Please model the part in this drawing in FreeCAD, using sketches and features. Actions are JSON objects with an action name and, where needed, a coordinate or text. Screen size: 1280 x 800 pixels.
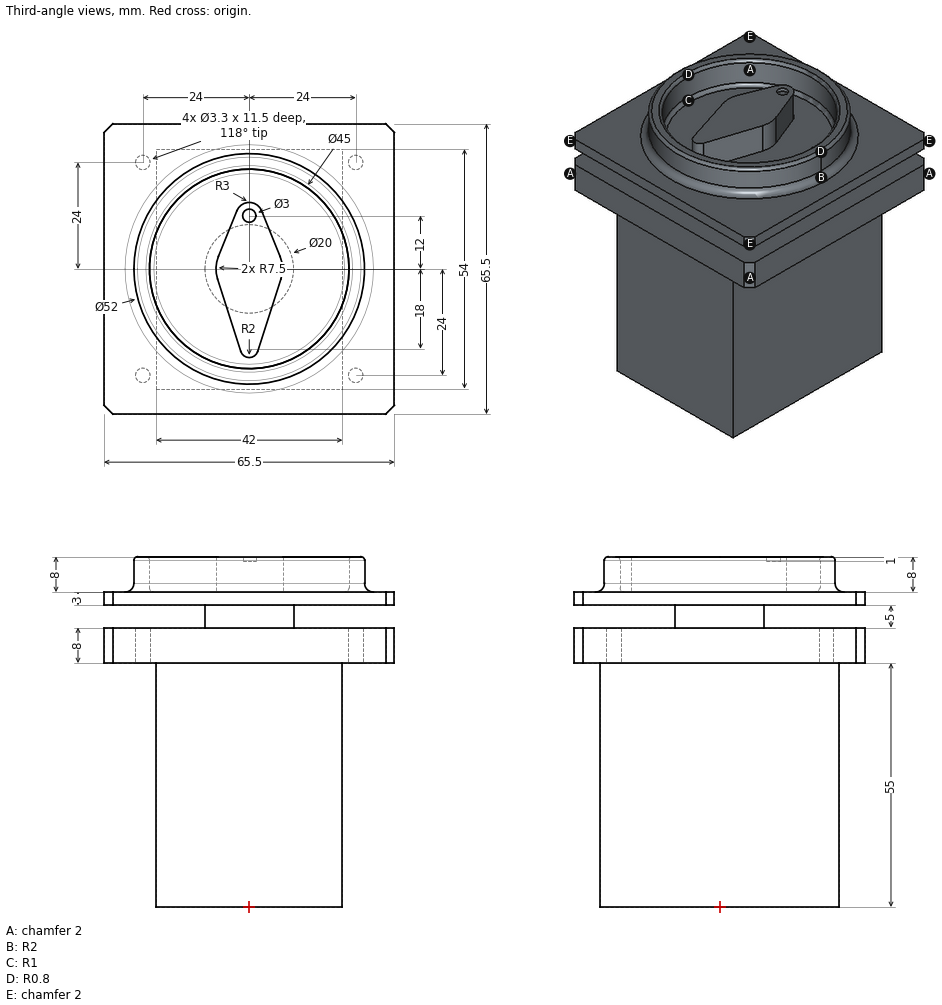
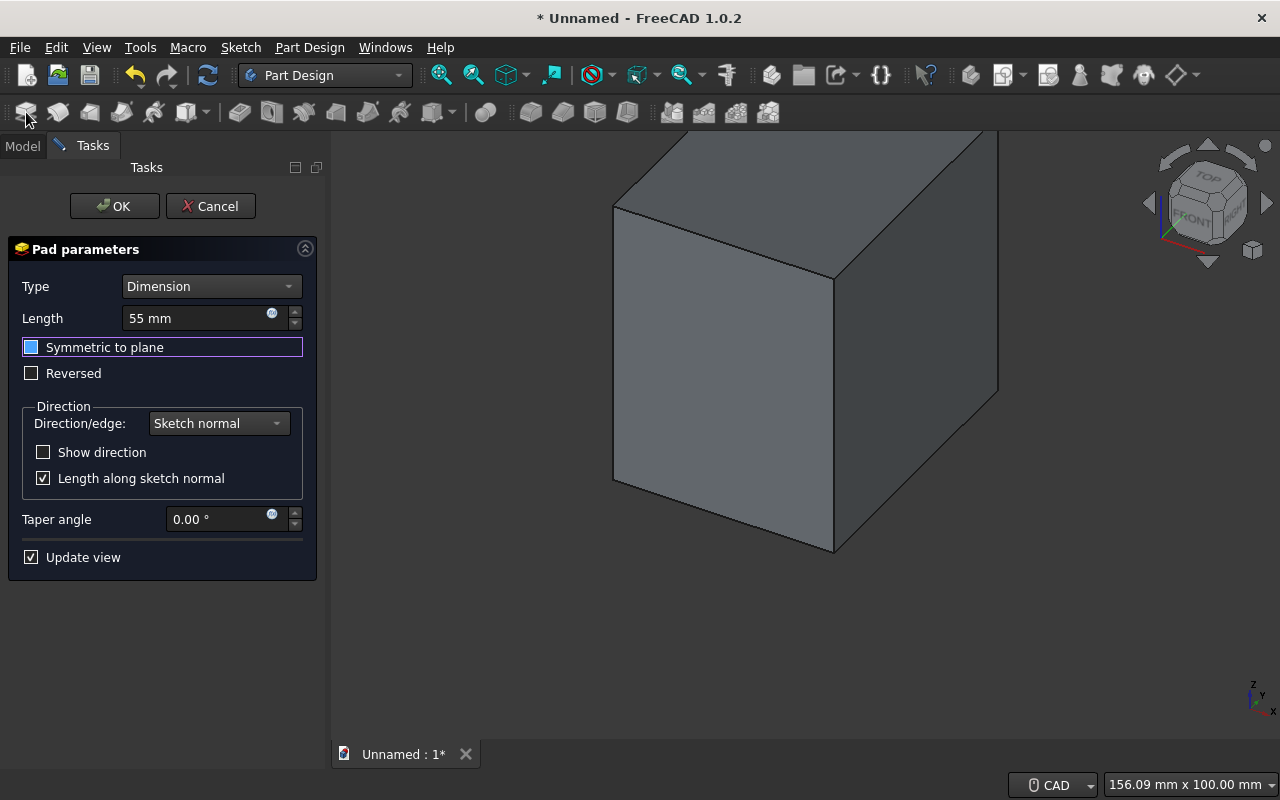
{"action": "left_click", "coordinate": [115, 206]}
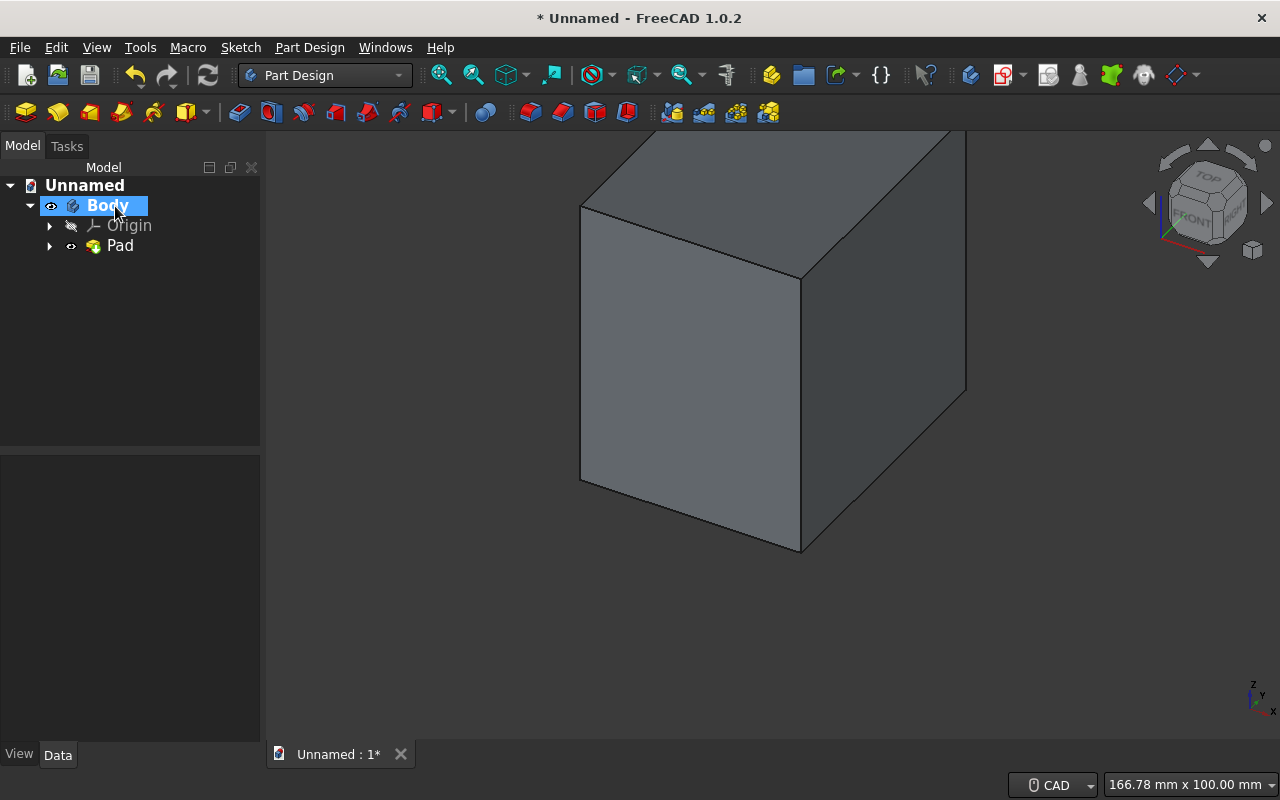
{"action": "left_click", "coordinate": [442, 76]}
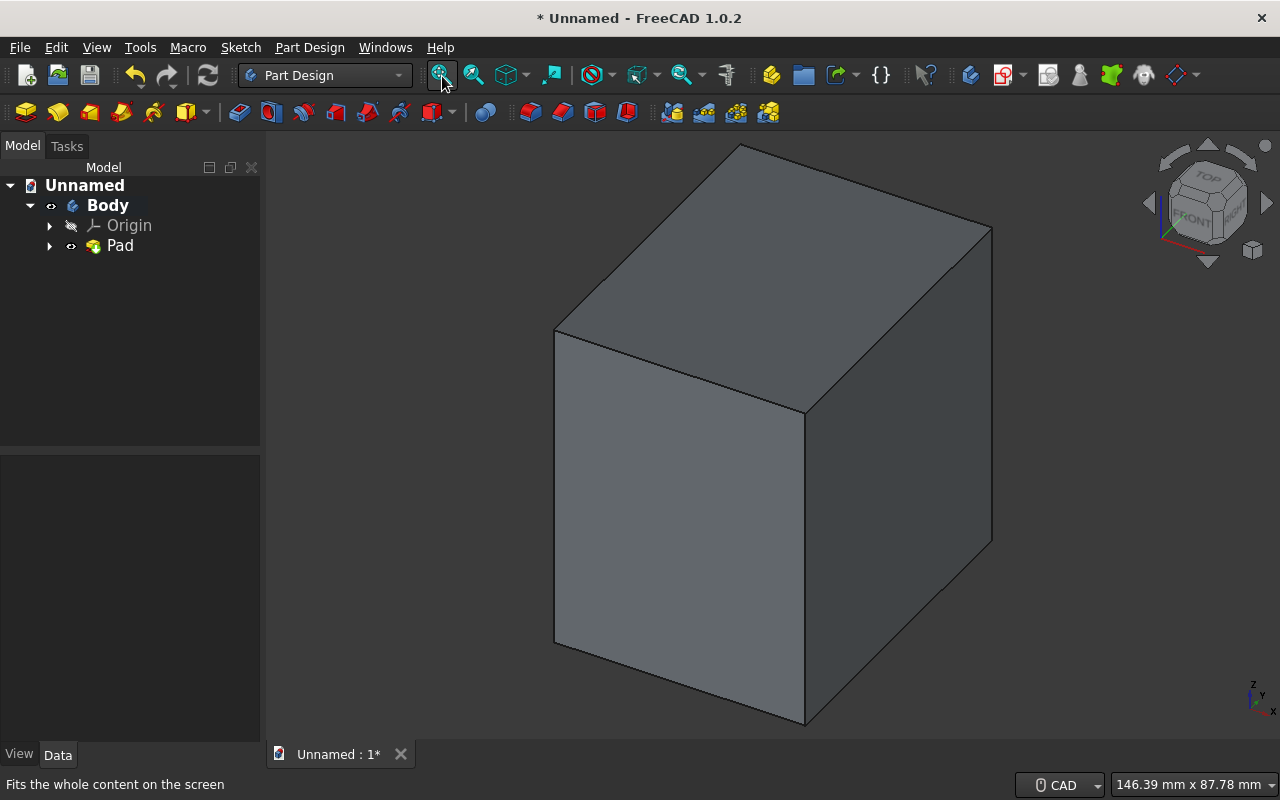
{"action": "left_click", "coordinate": [773, 278]}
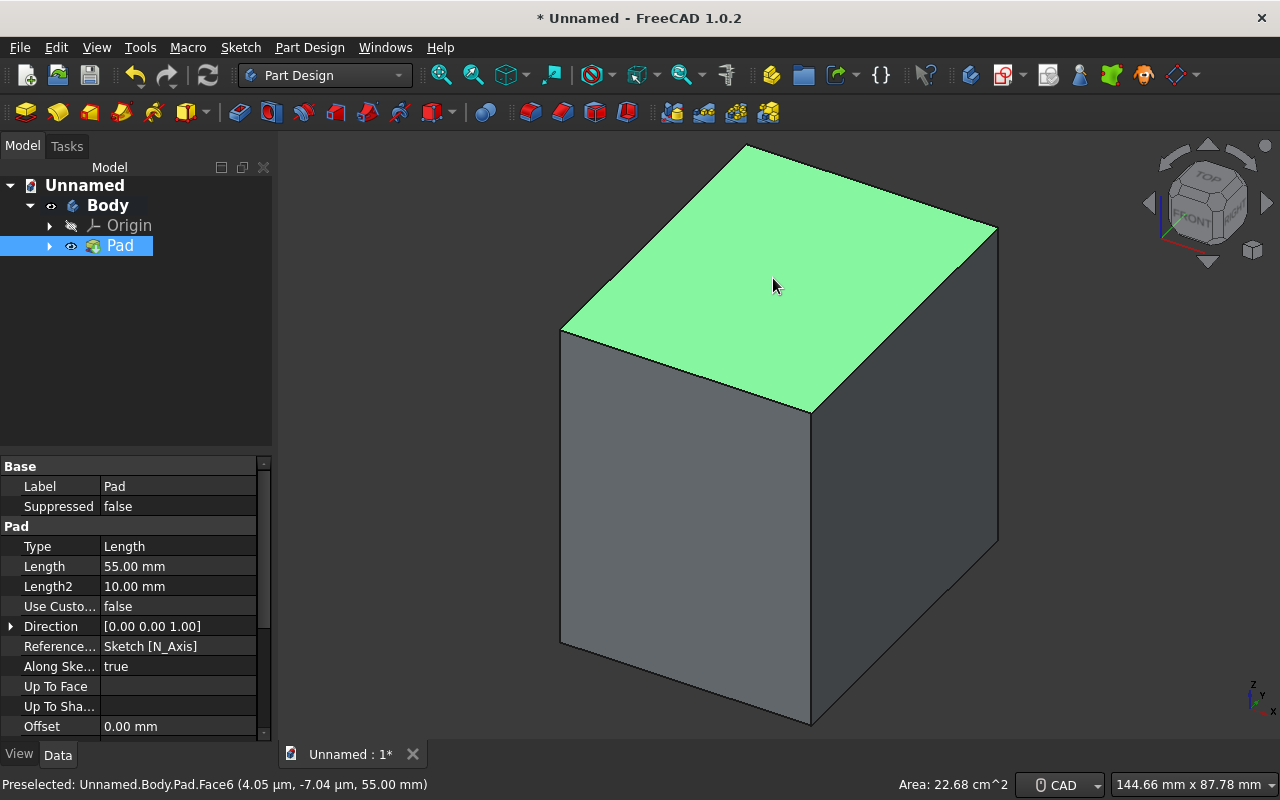
{"action": "left_click", "coordinate": [1004, 76]}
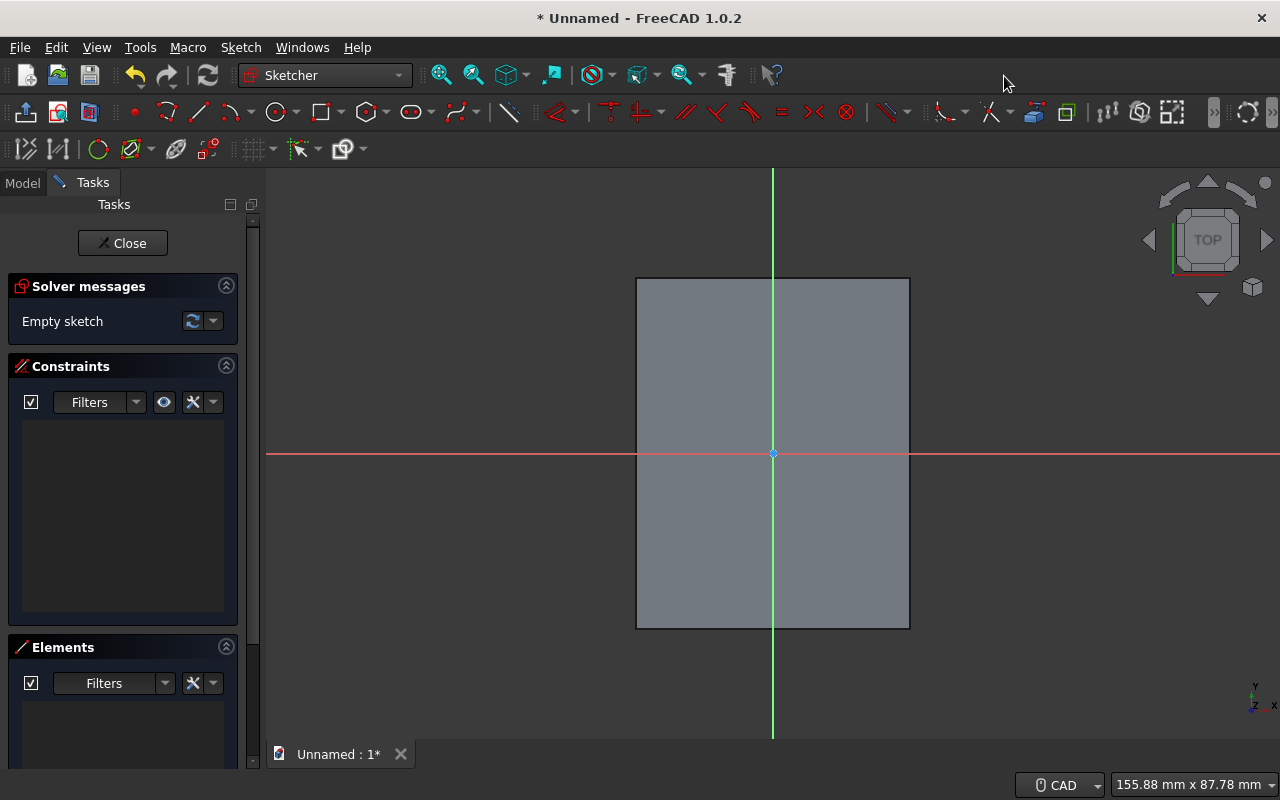
{"action": "left_click", "coordinate": [344, 112]}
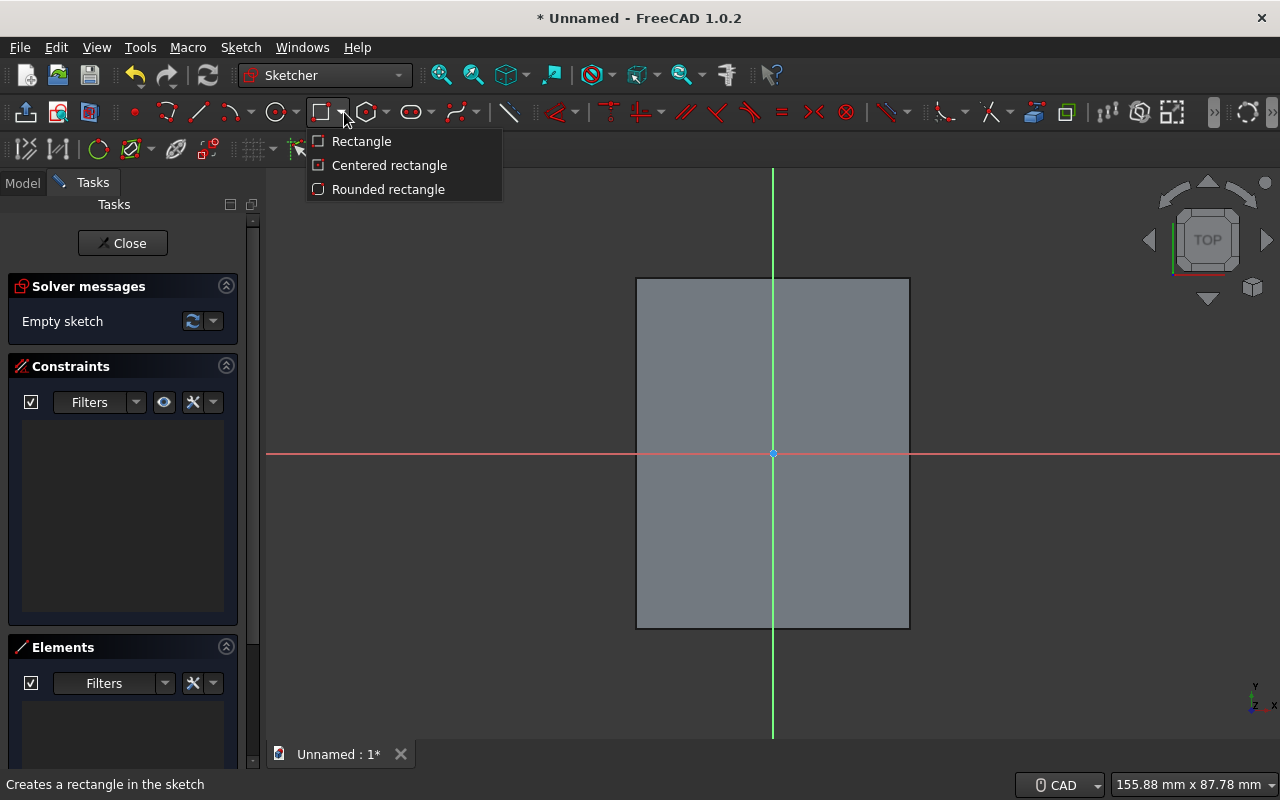
{"action": "left_click", "coordinate": [404, 165]}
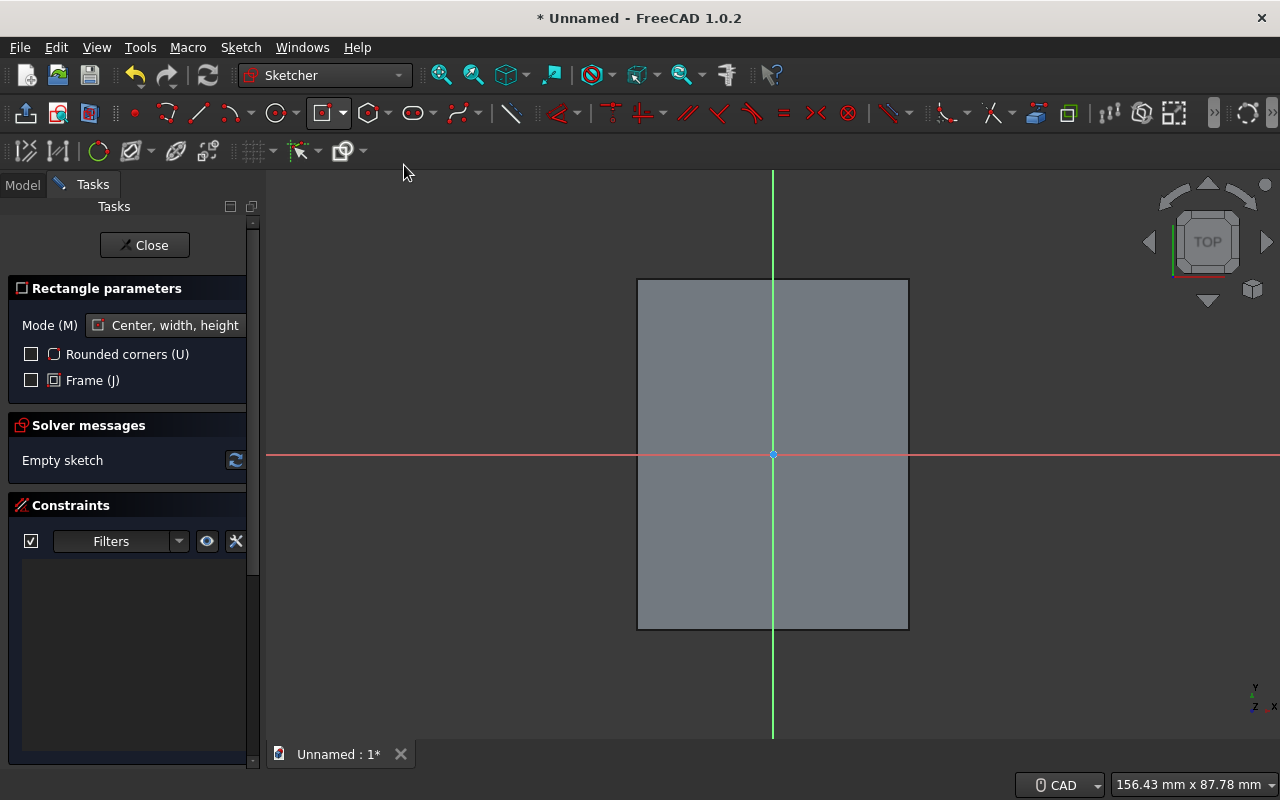
{"action": "left_click", "coordinate": [773, 454]}
{"action": "mouse_move", "coordinate": [985, 242]}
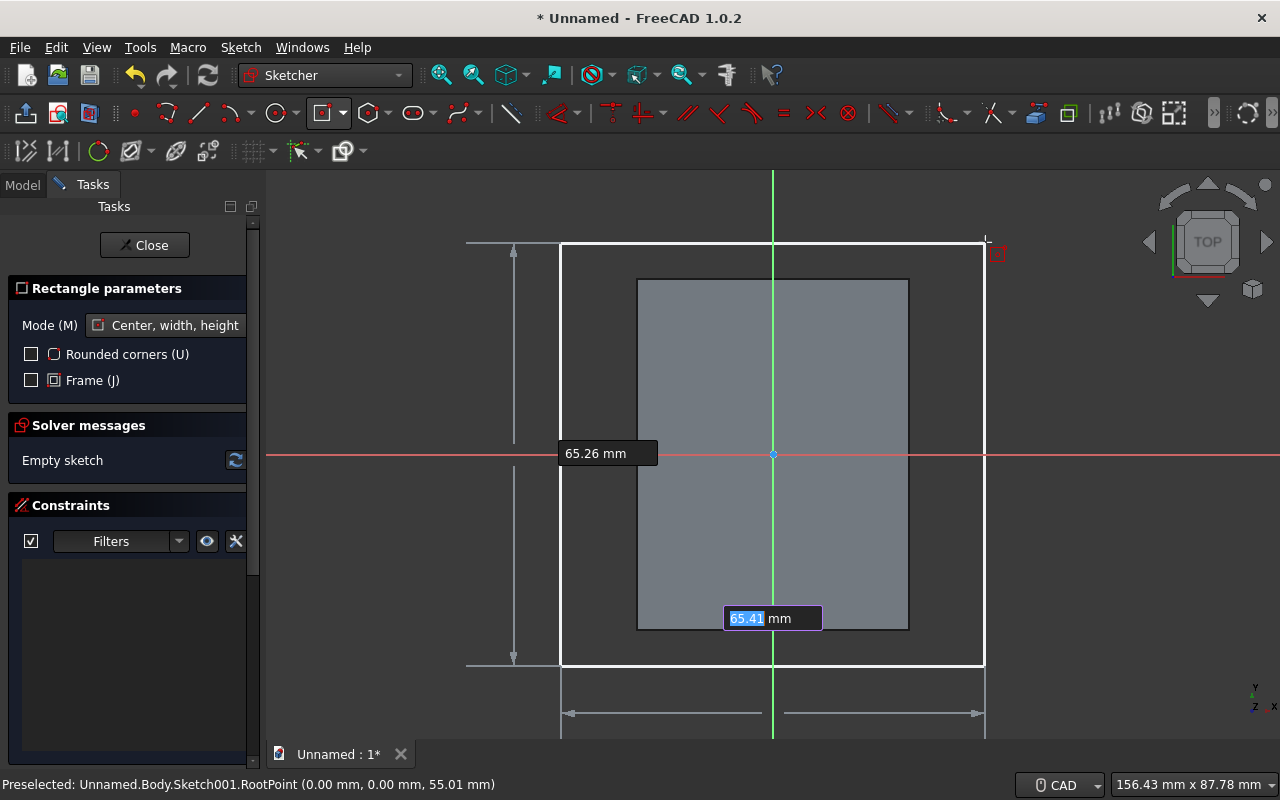
{"action": "type", "text": "65.5"}
{"action": "key", "text": "Tab"}
{"action": "type", "text": "65.5"}
{"action": "key", "text": "Return"}
{"action": "key", "text": "Escape"}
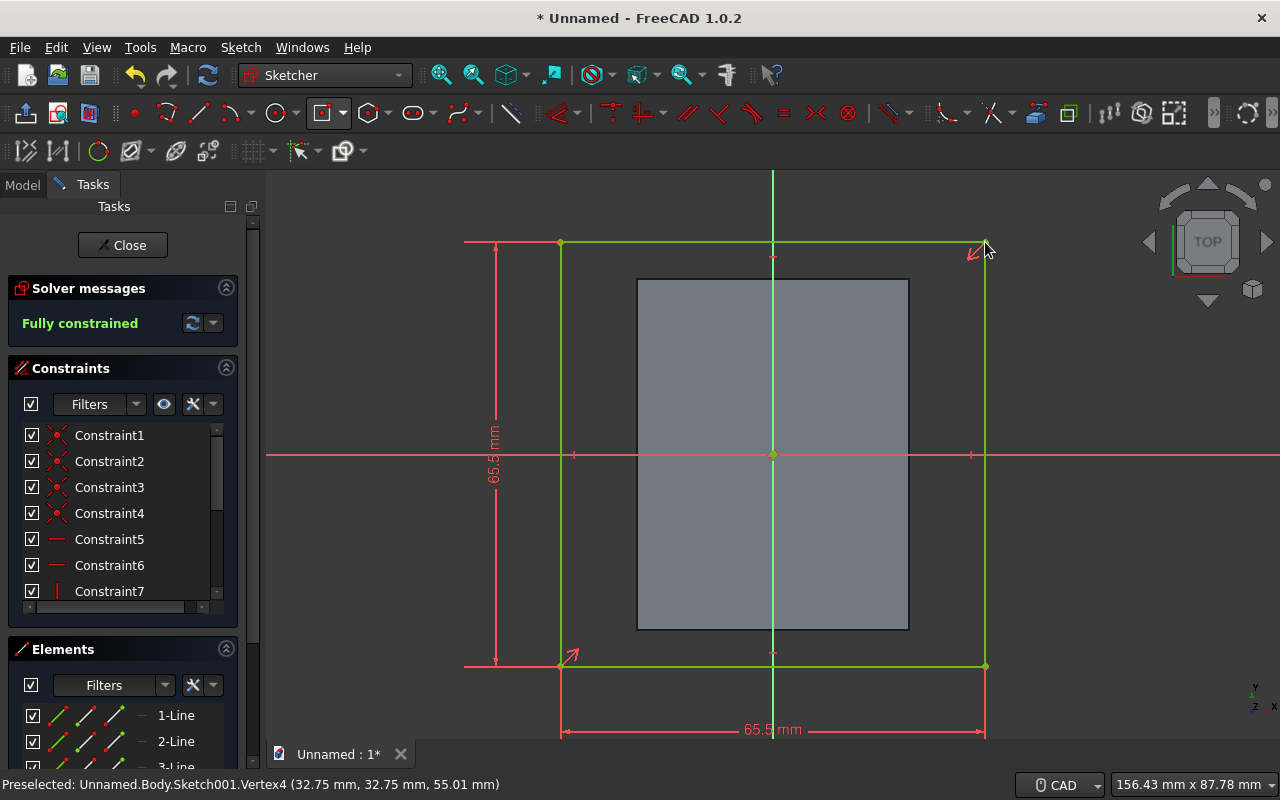
{"action": "left_click", "coordinate": [123, 245]}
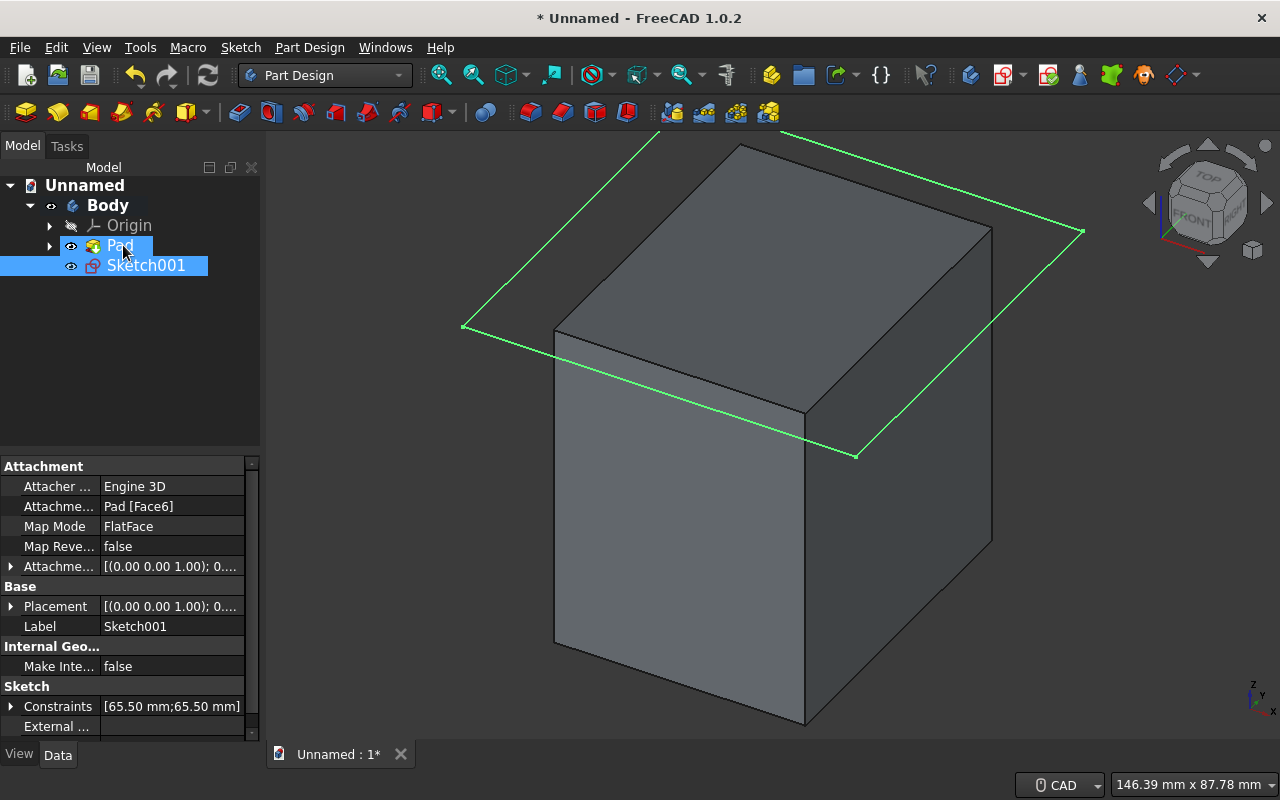
{"action": "left_click", "coordinate": [26, 112]}